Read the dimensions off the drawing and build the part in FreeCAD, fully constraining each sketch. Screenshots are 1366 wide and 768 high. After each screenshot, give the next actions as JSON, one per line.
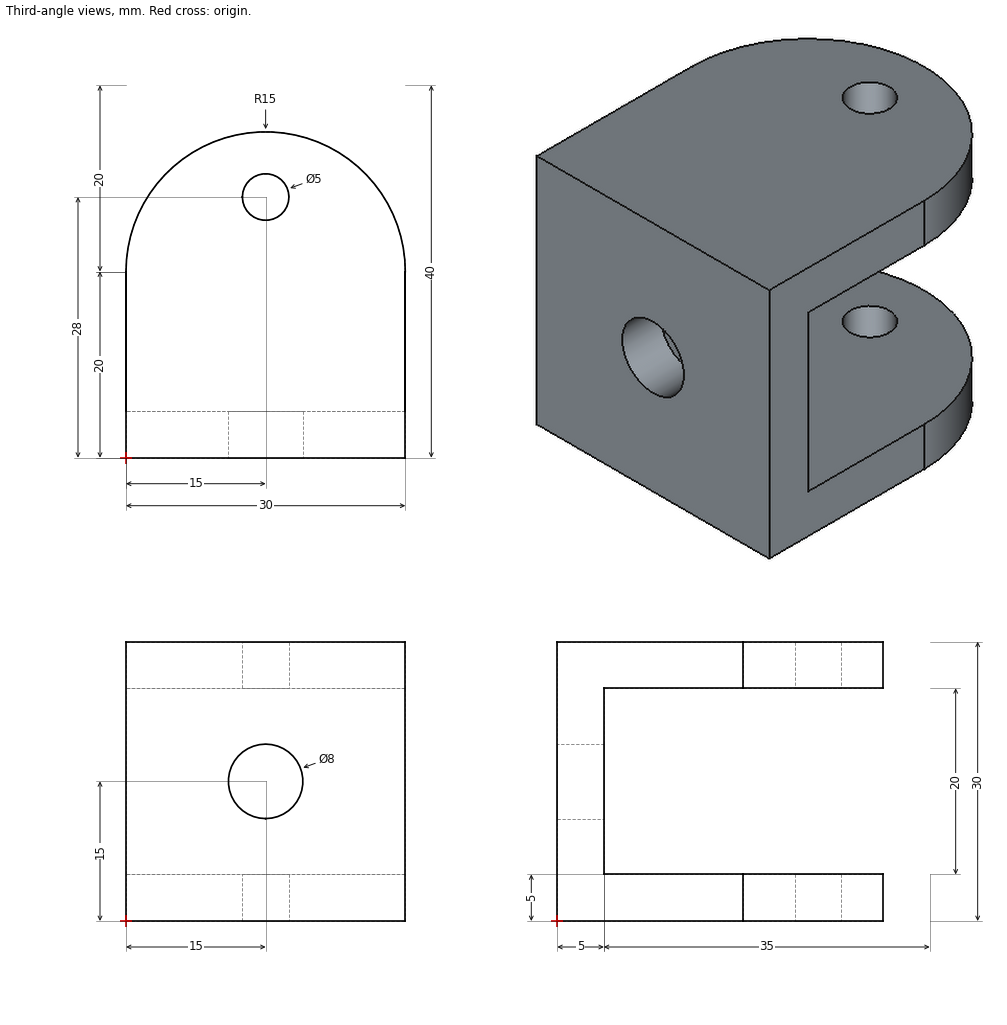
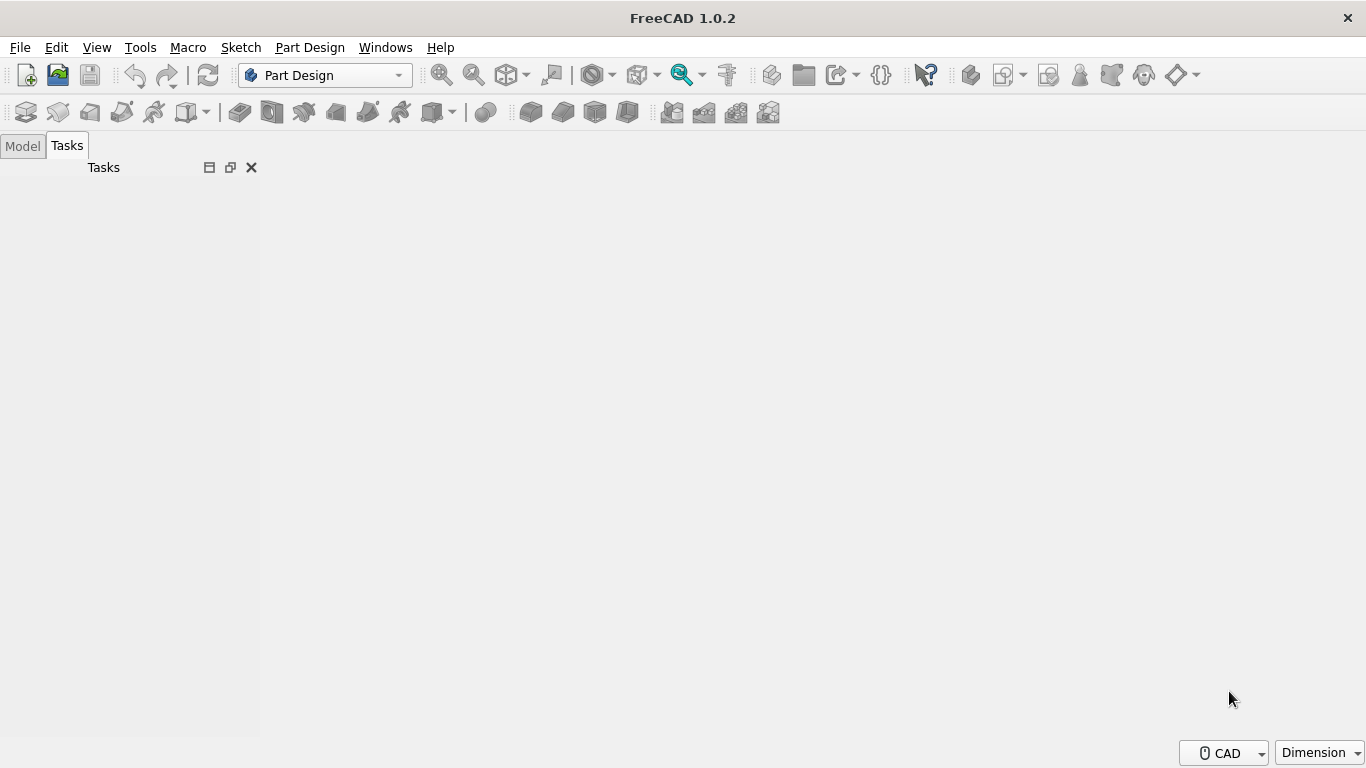
{"action": "left_click", "coordinate": [26, 76]}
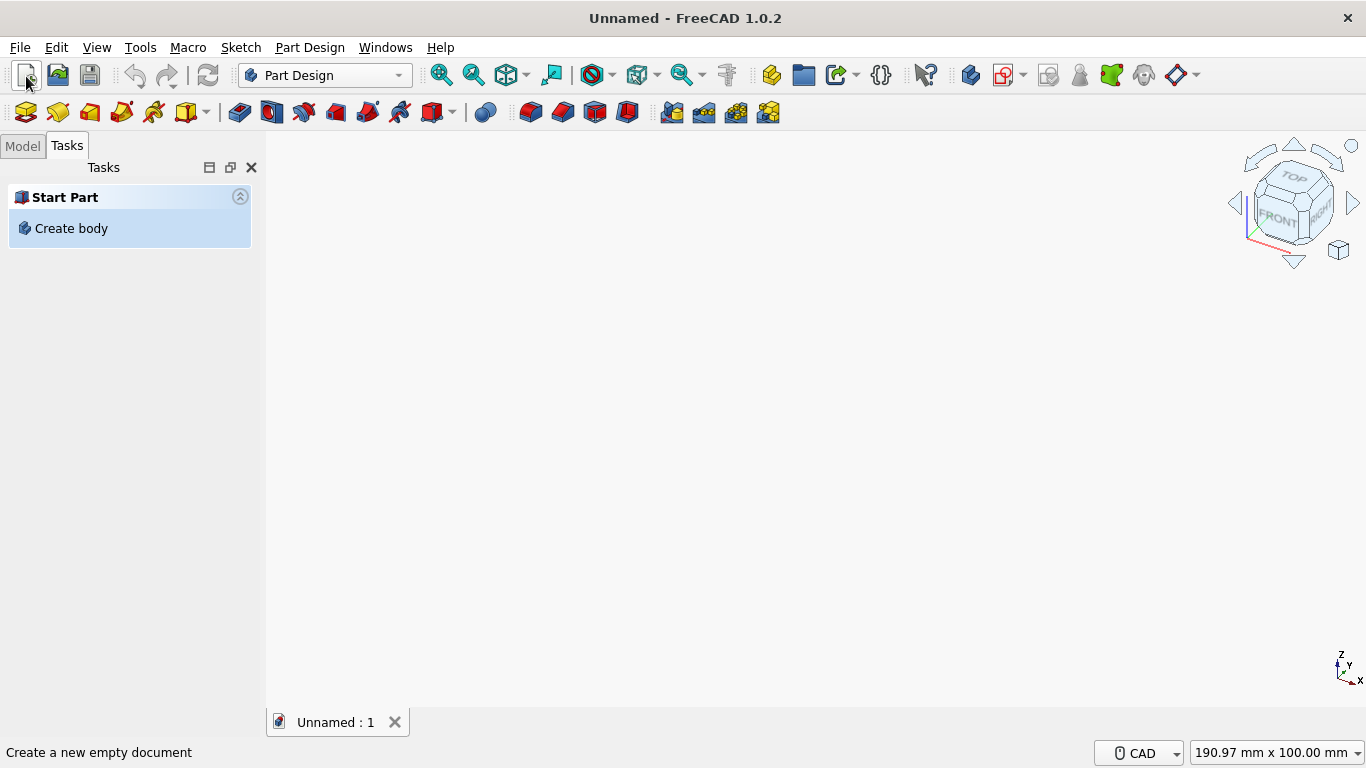
{"action": "left_click", "coordinate": [1004, 76]}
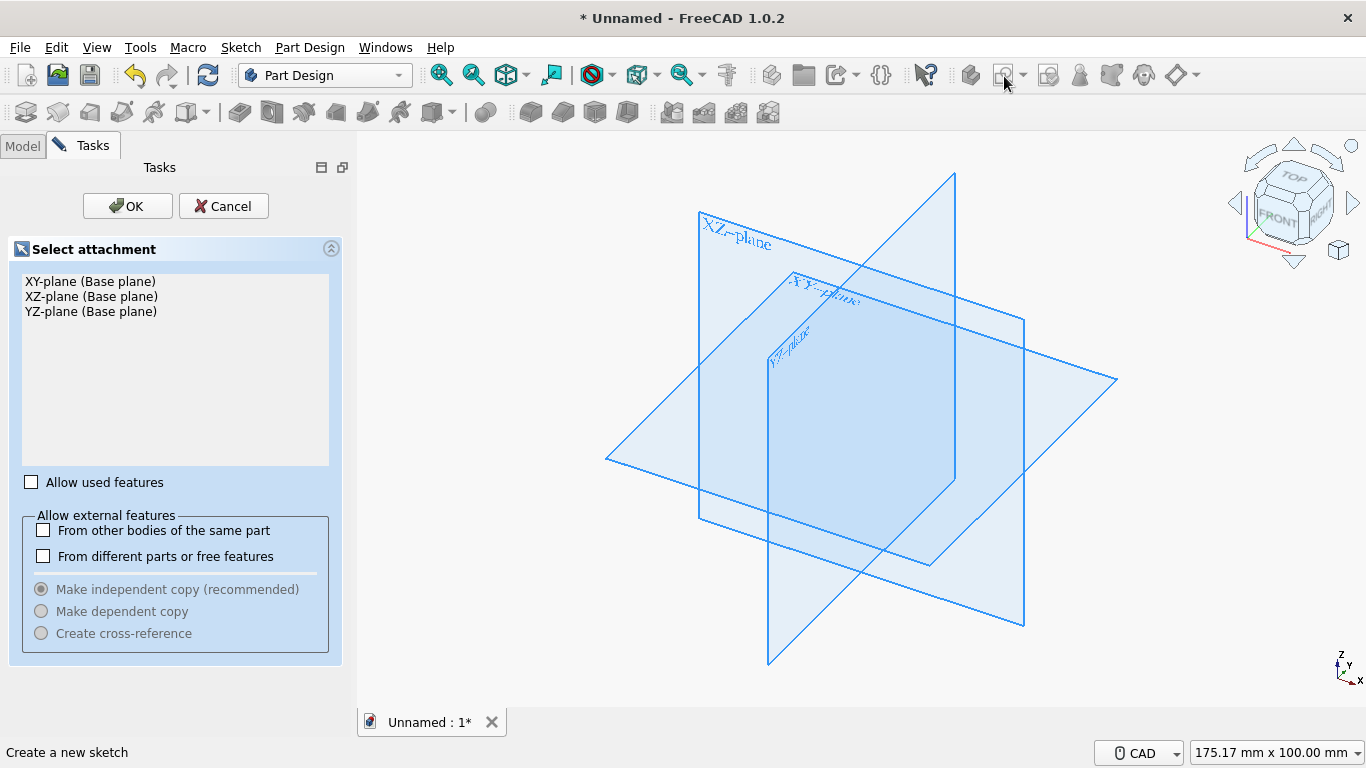
{"action": "left_click", "coordinate": [82, 282]}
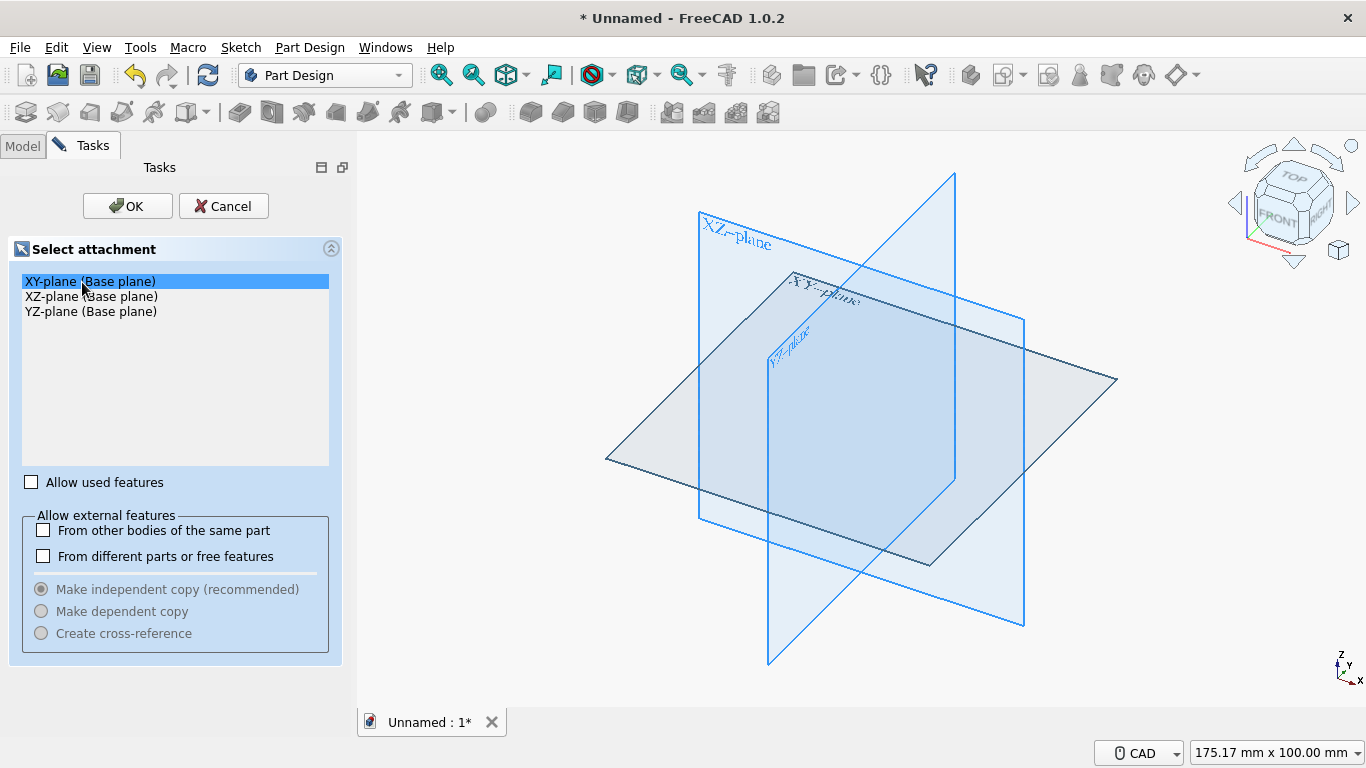
{"action": "left_click", "coordinate": [128, 206]}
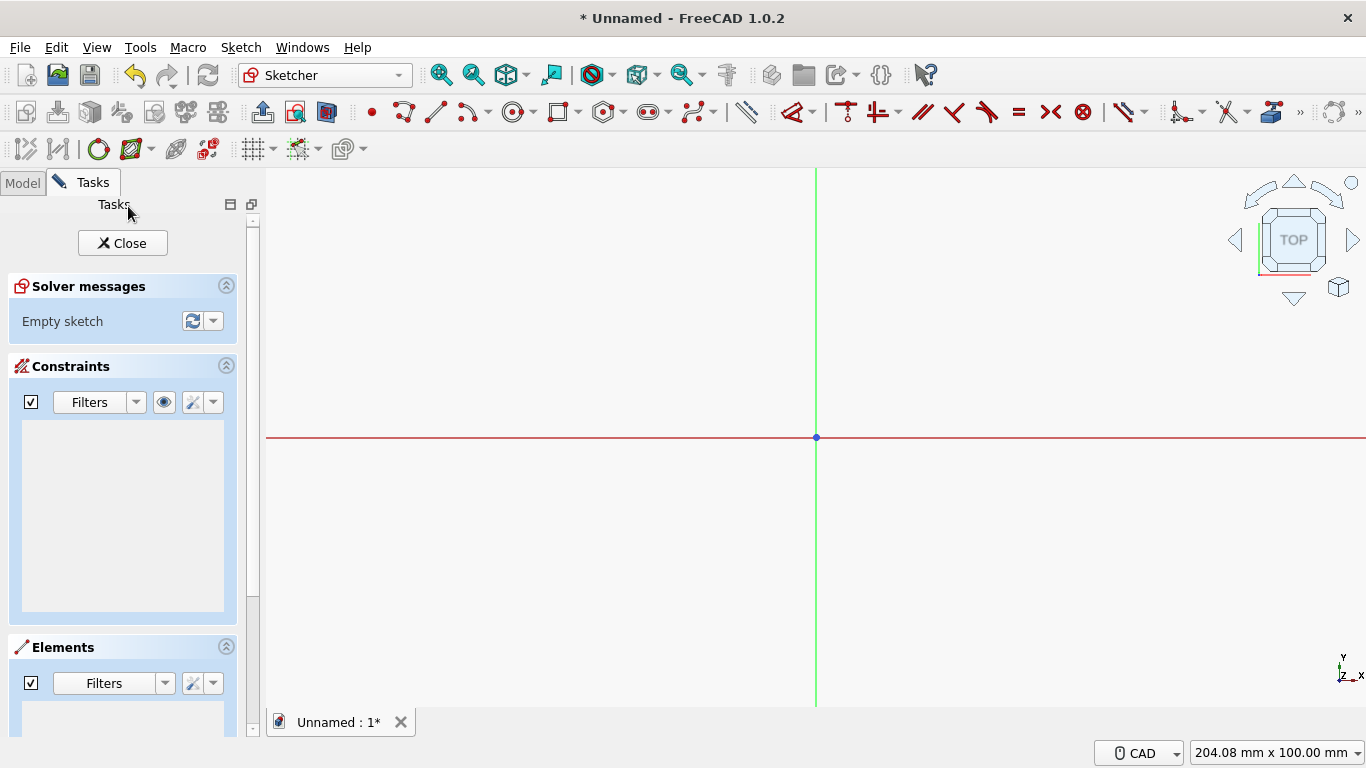
{"action": "scroll", "coordinate": [1201, 196], "scroll_direction": "up", "scroll_amount": 2}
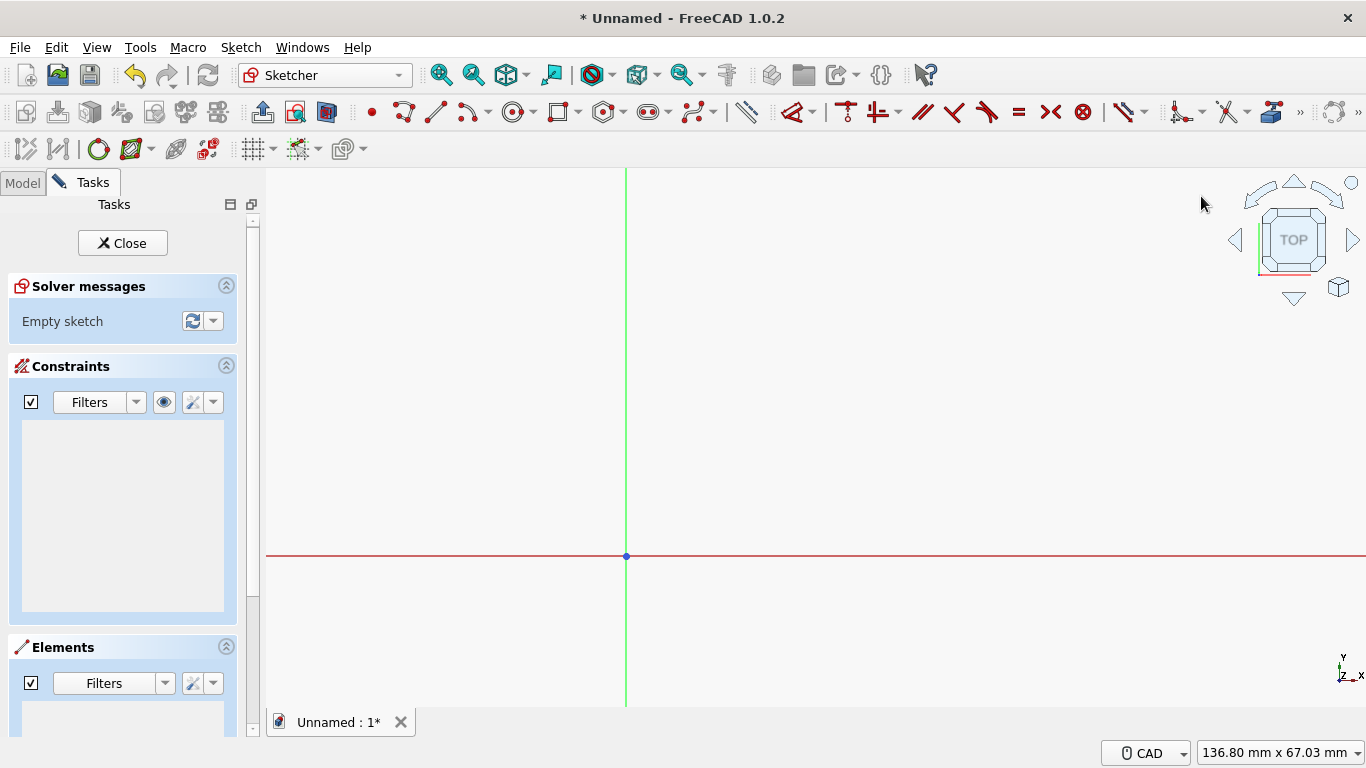
{"action": "left_click", "coordinate": [558, 112]}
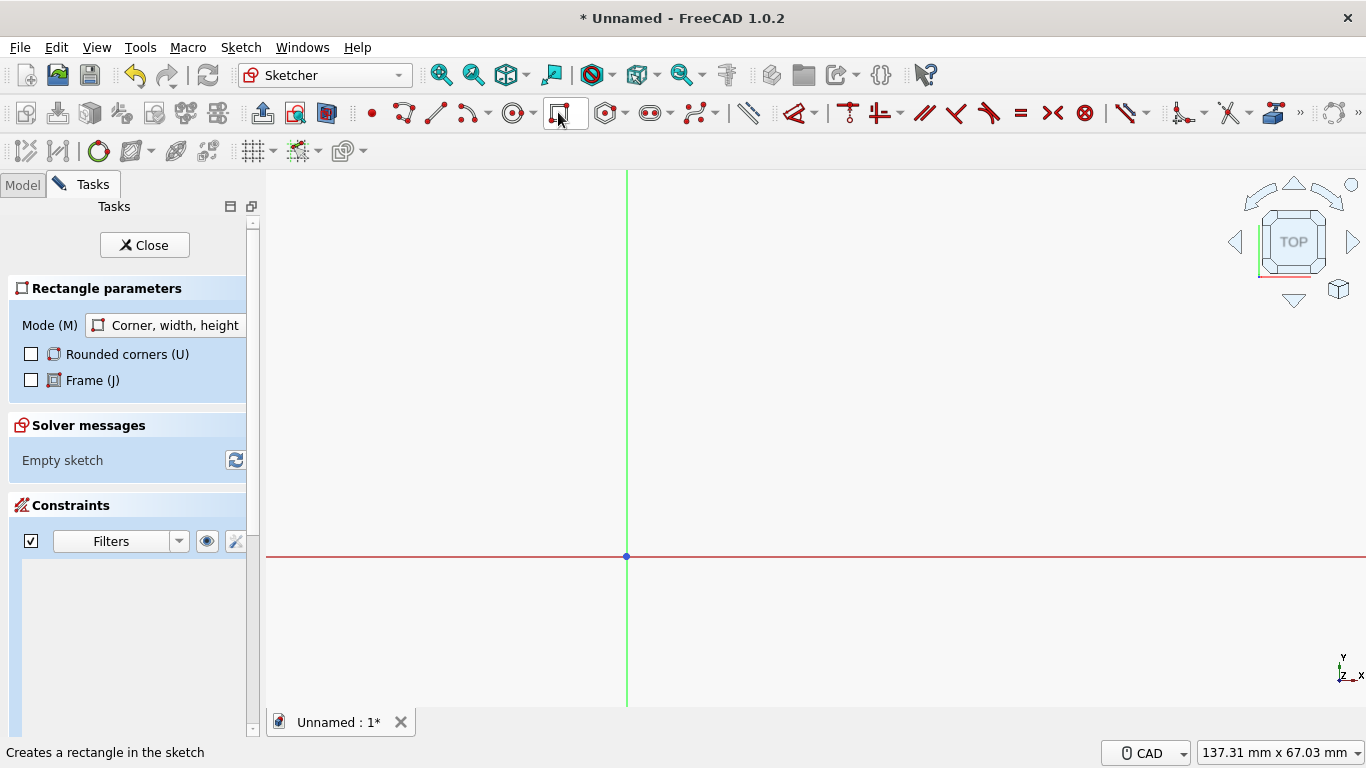
{"action": "left_click", "coordinate": [627, 557]}
{"action": "mouse_move", "coordinate": [867, 236]}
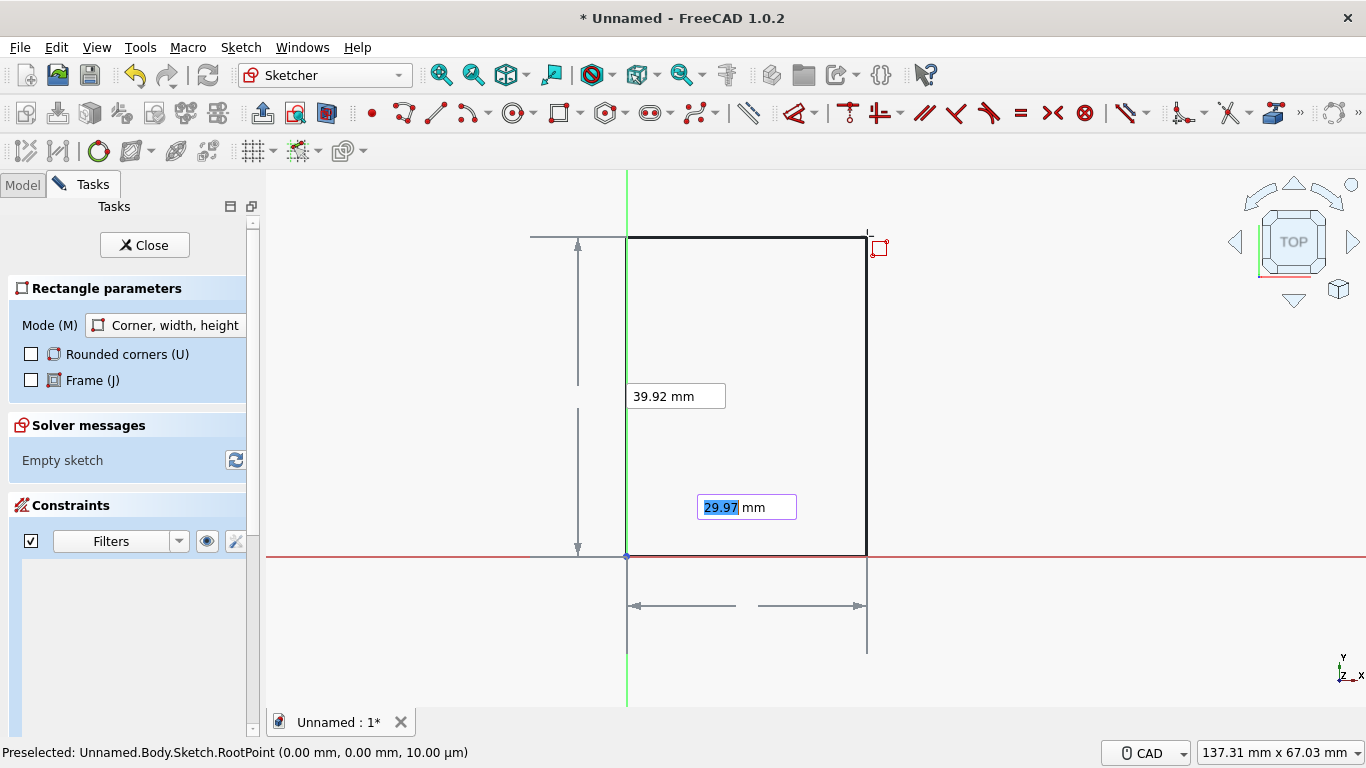
{"action": "type", "text": "30"}
{"action": "key", "text": "Tab"}
{"action": "type", "text": "40"}
{"action": "key", "text": "Return"}
{"action": "key", "text": "Escape"}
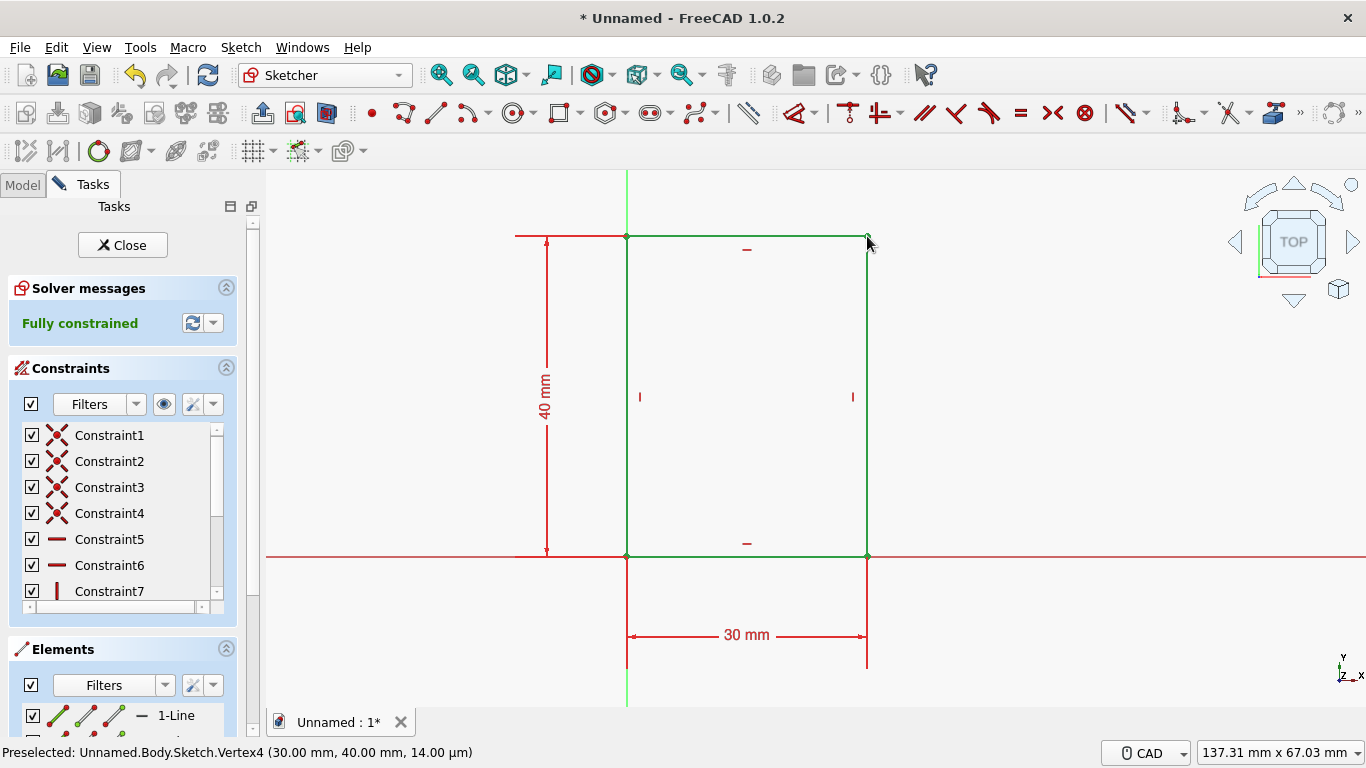
{"action": "left_click", "coordinate": [123, 245]}